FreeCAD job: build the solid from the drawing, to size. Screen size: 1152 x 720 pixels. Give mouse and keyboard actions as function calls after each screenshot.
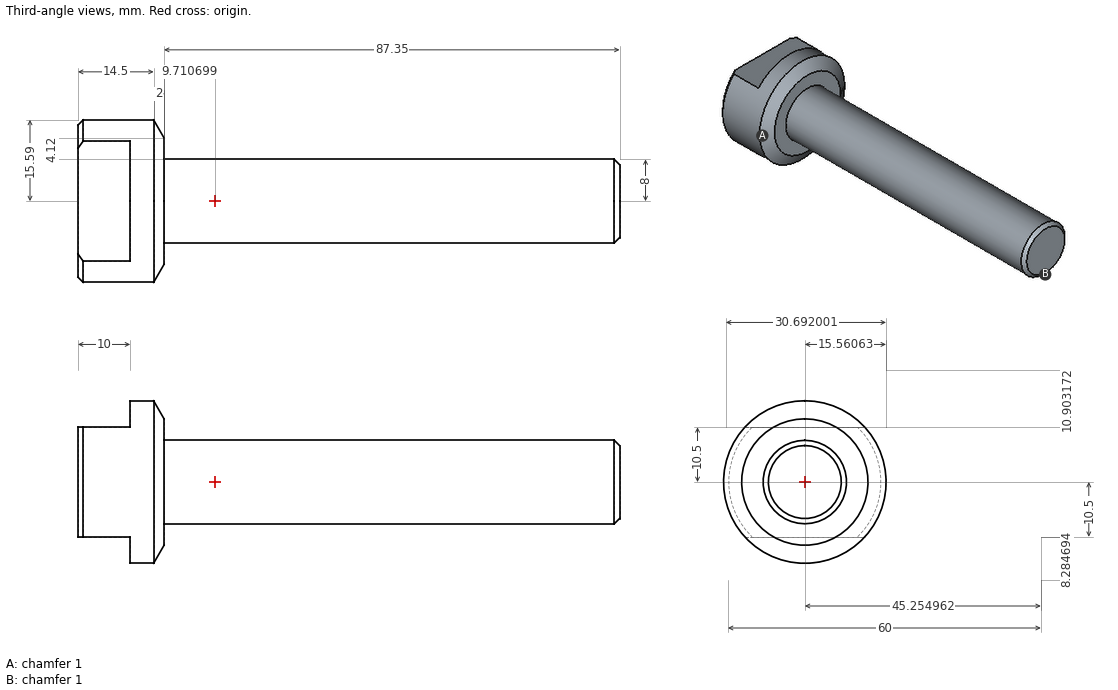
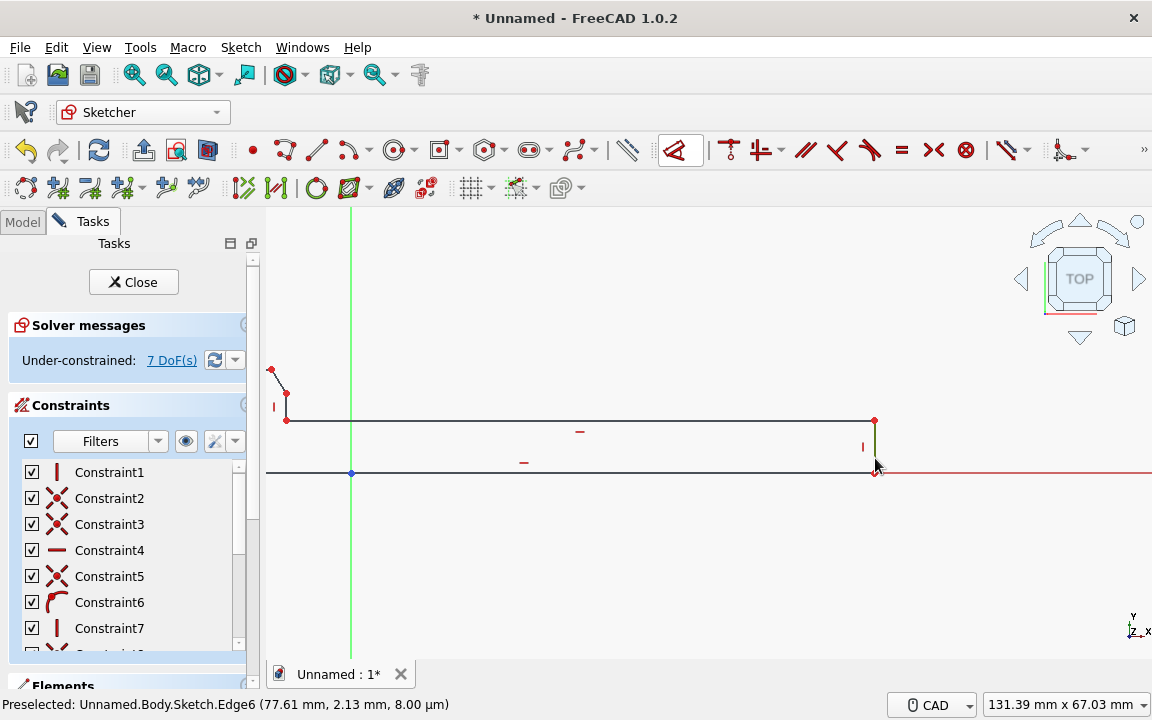
key(i)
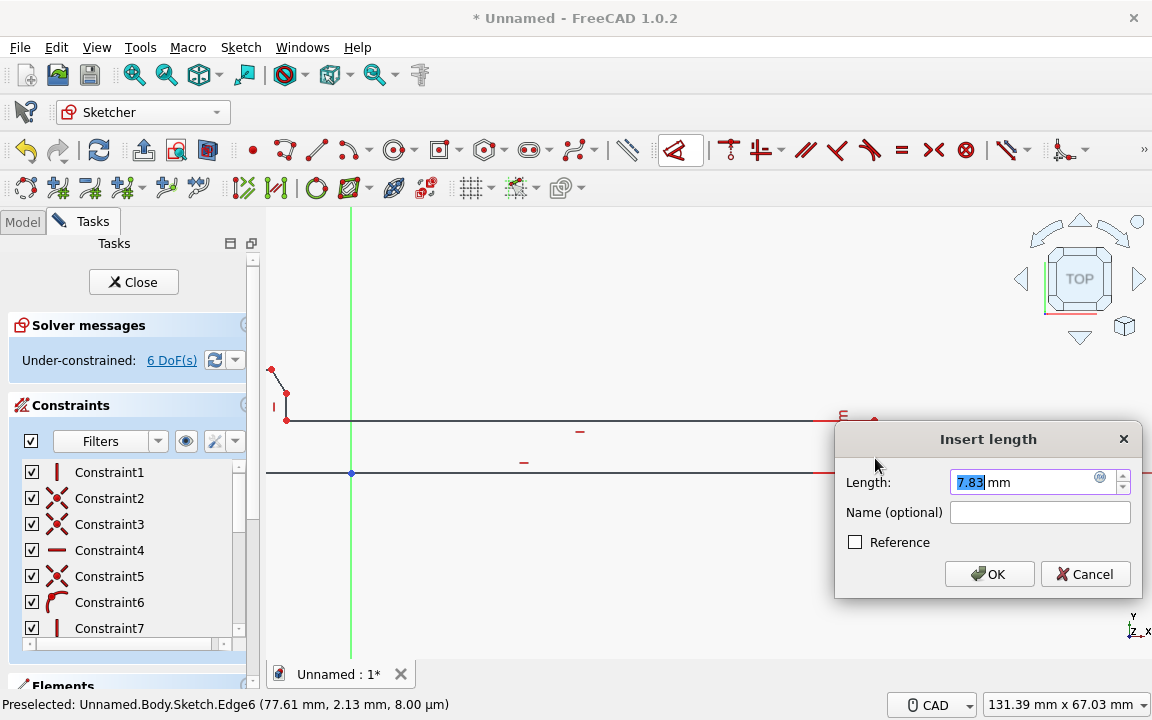
text(8)
key(Return)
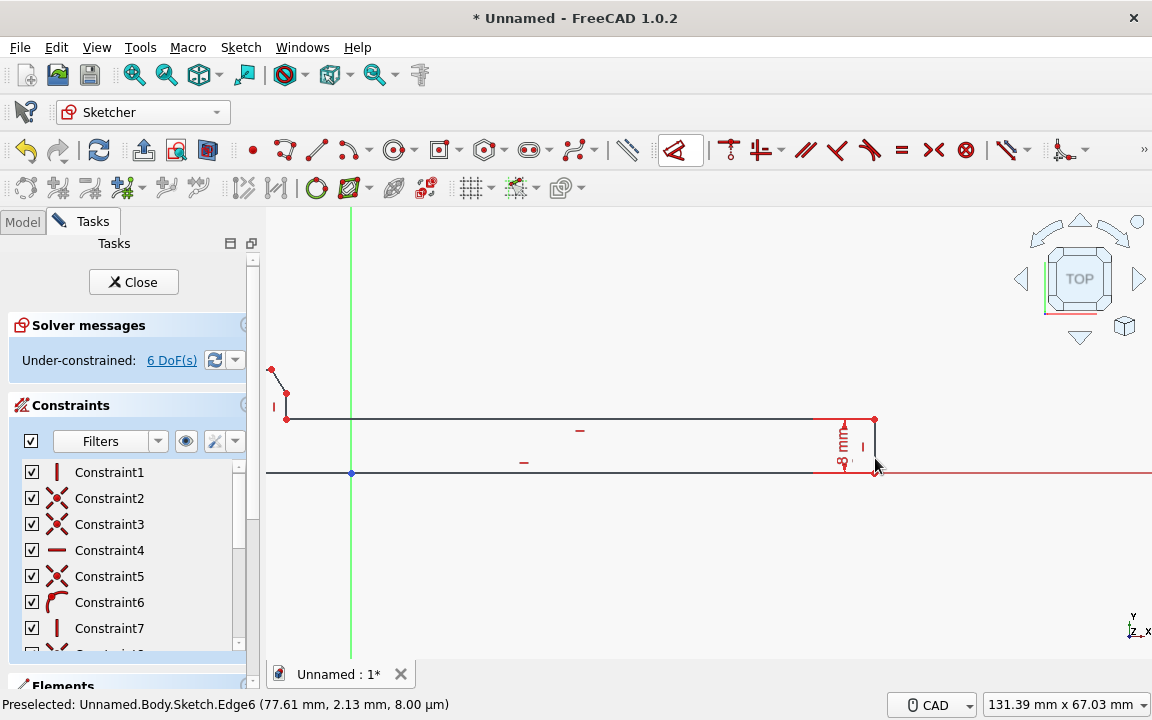
scroll(876, 458, down, 2)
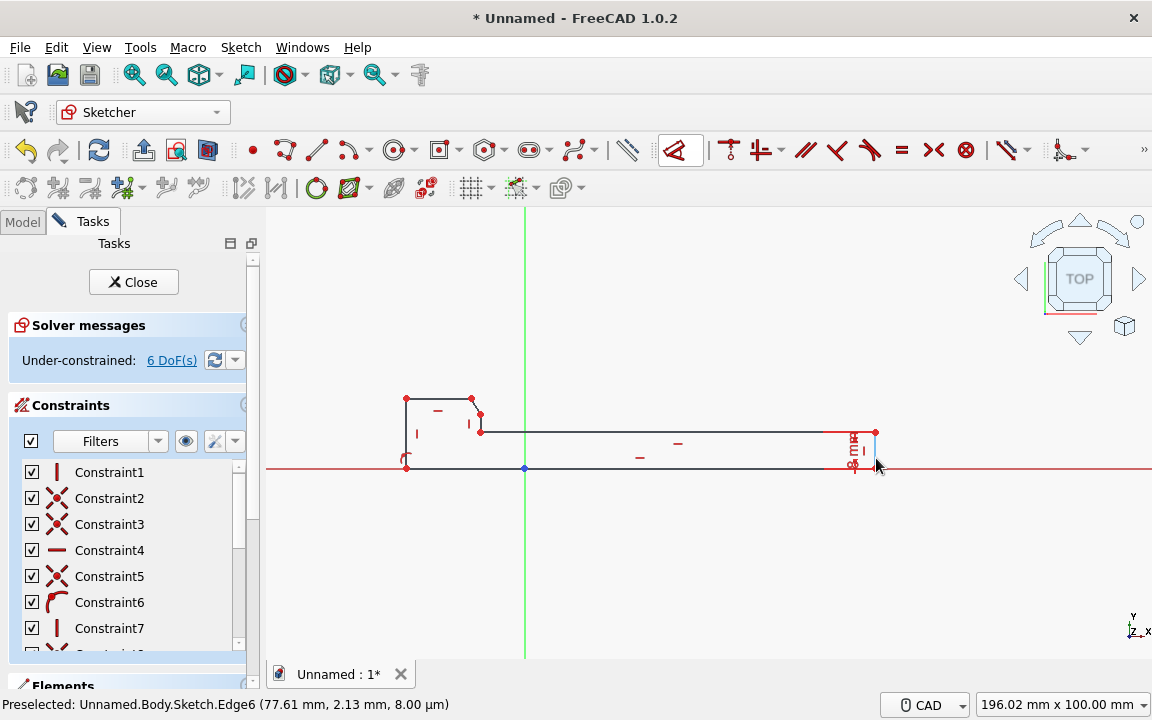
scroll(477, 408, up, 8)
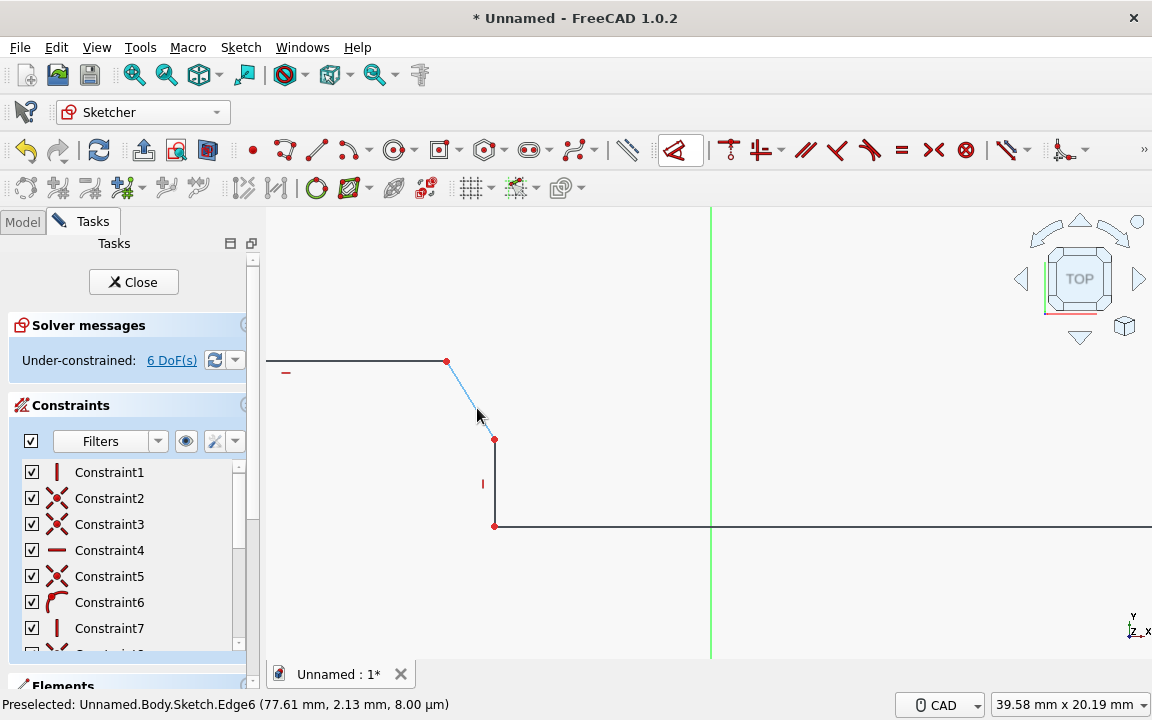
click(476, 408)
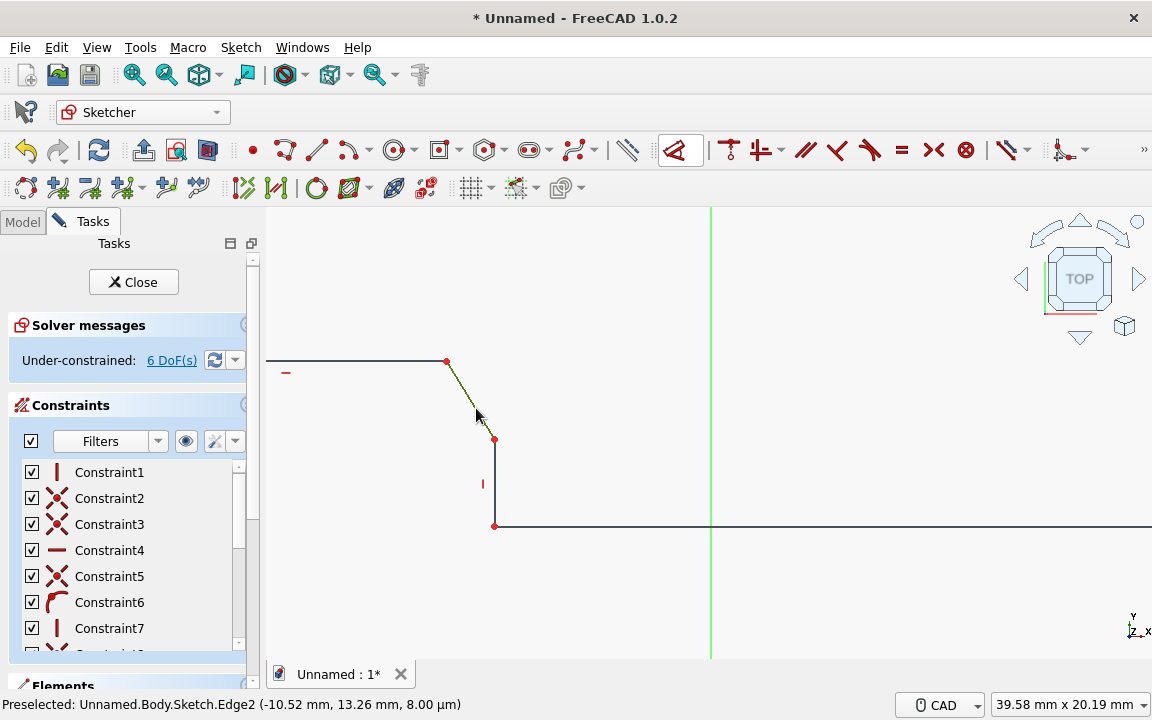
key(l)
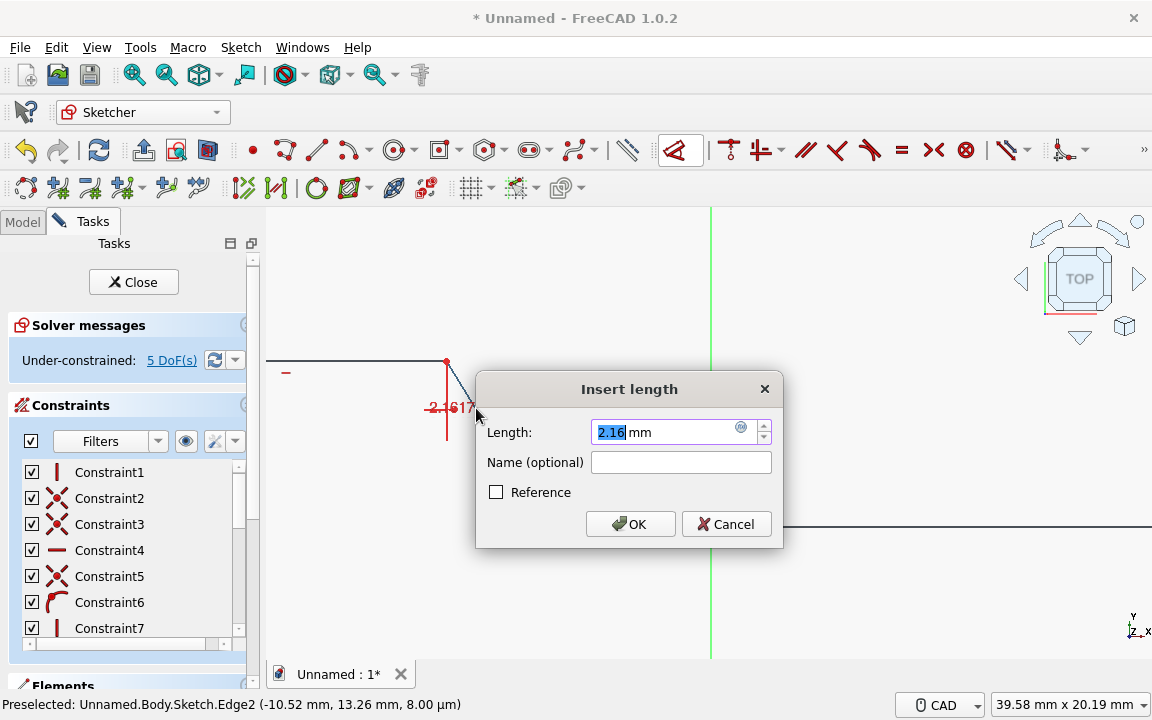
text(2)
key(Return)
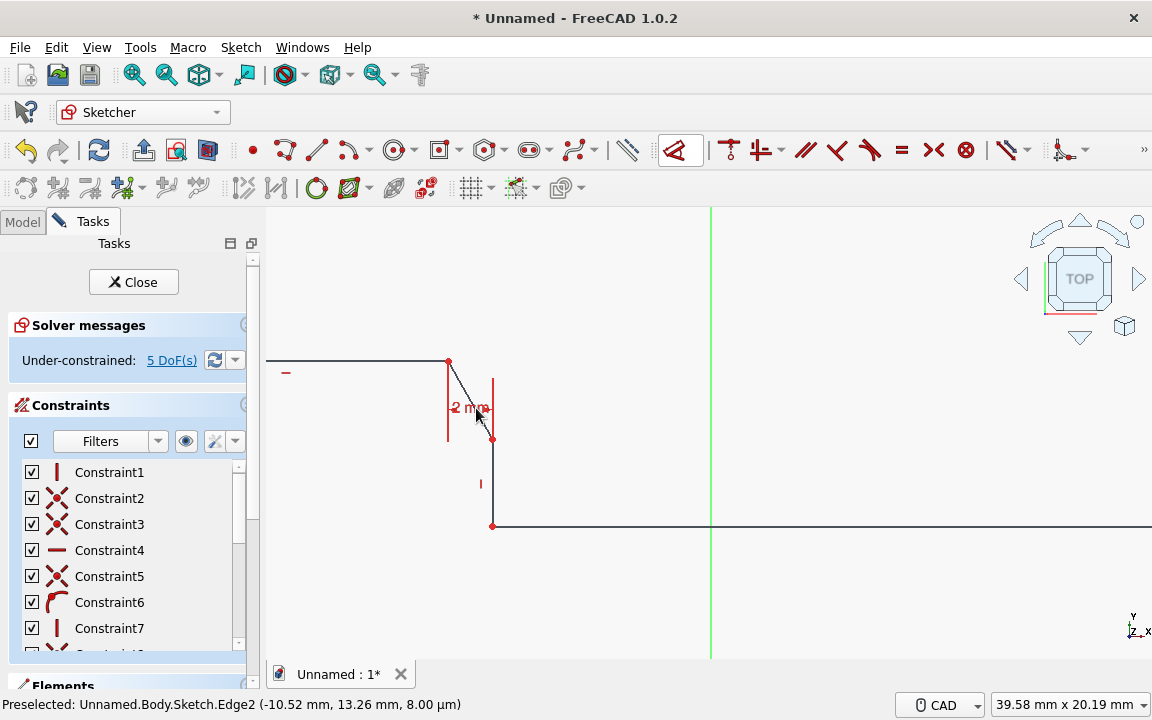
click(493, 501)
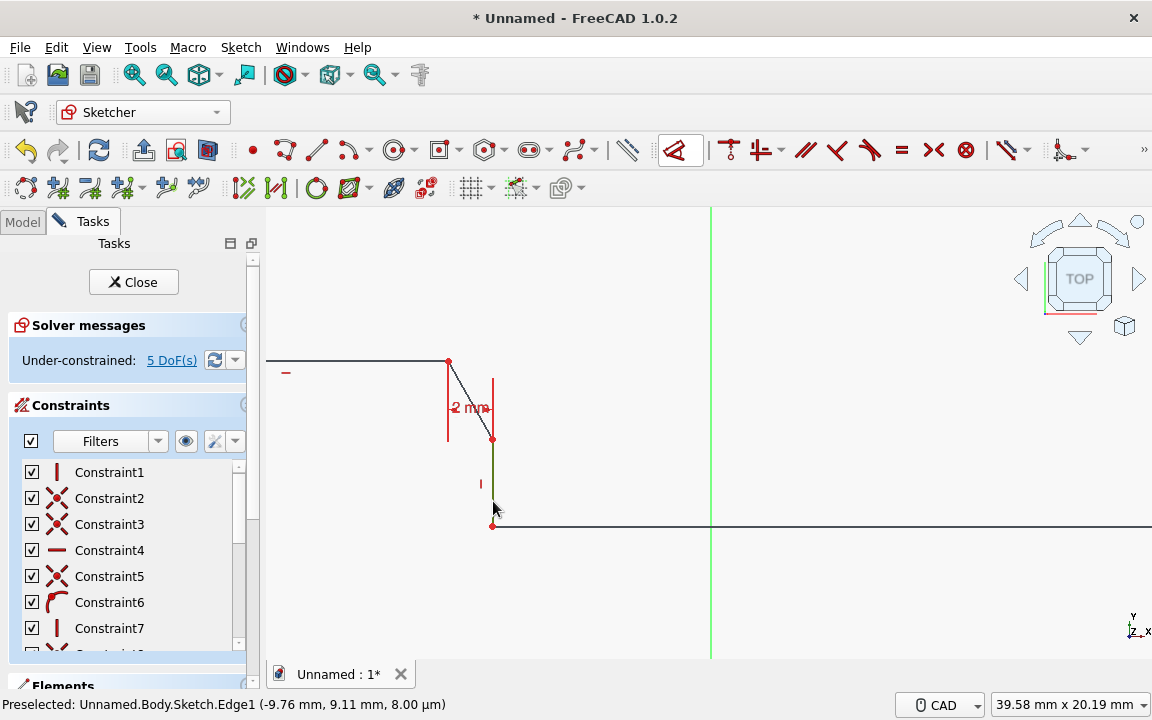
key(i)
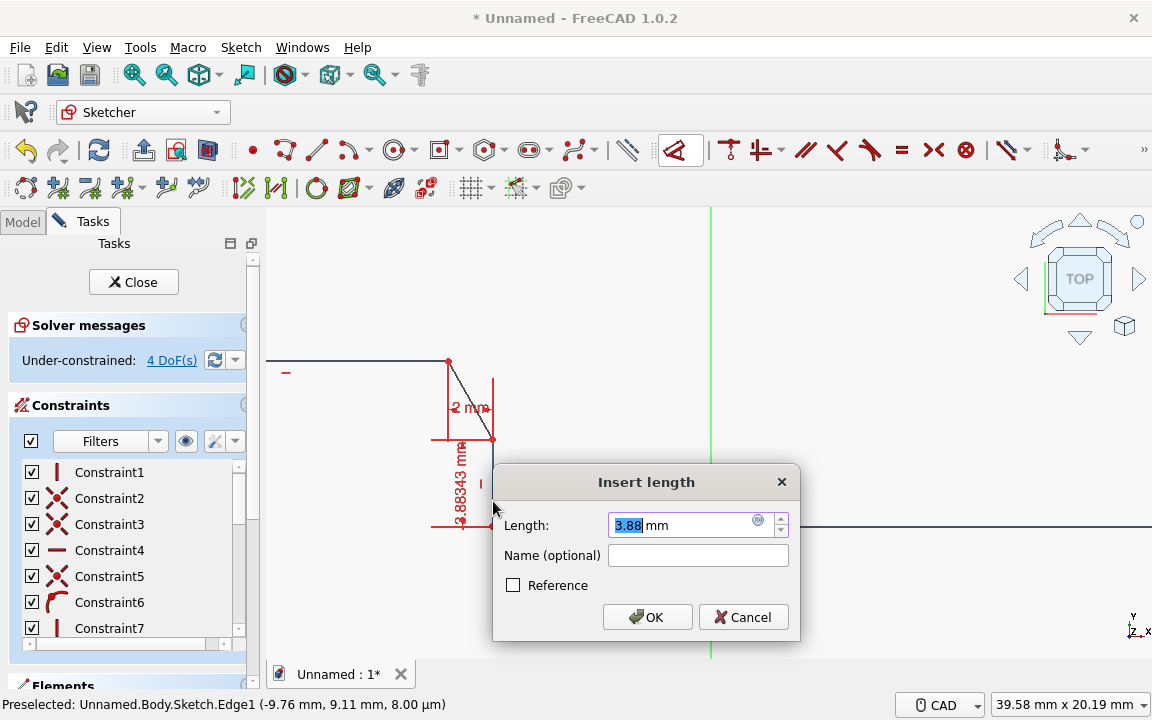
text(4.12)
key(Return)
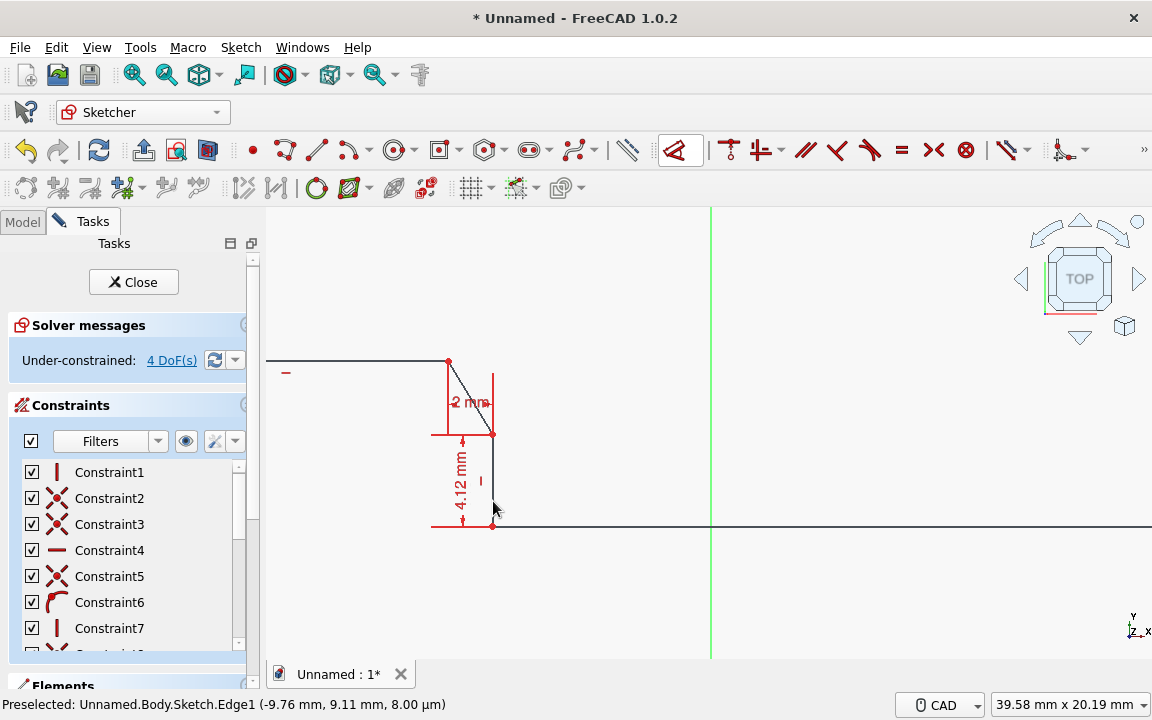
scroll(477, 408, down, 8)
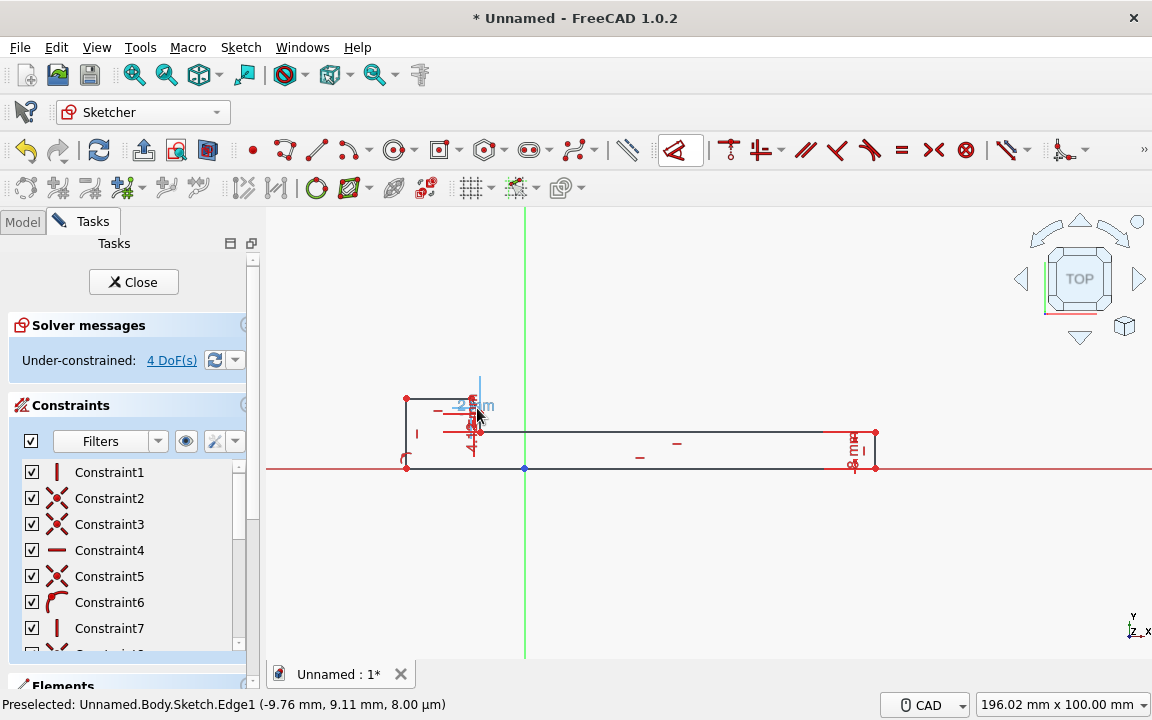
click(452, 399)